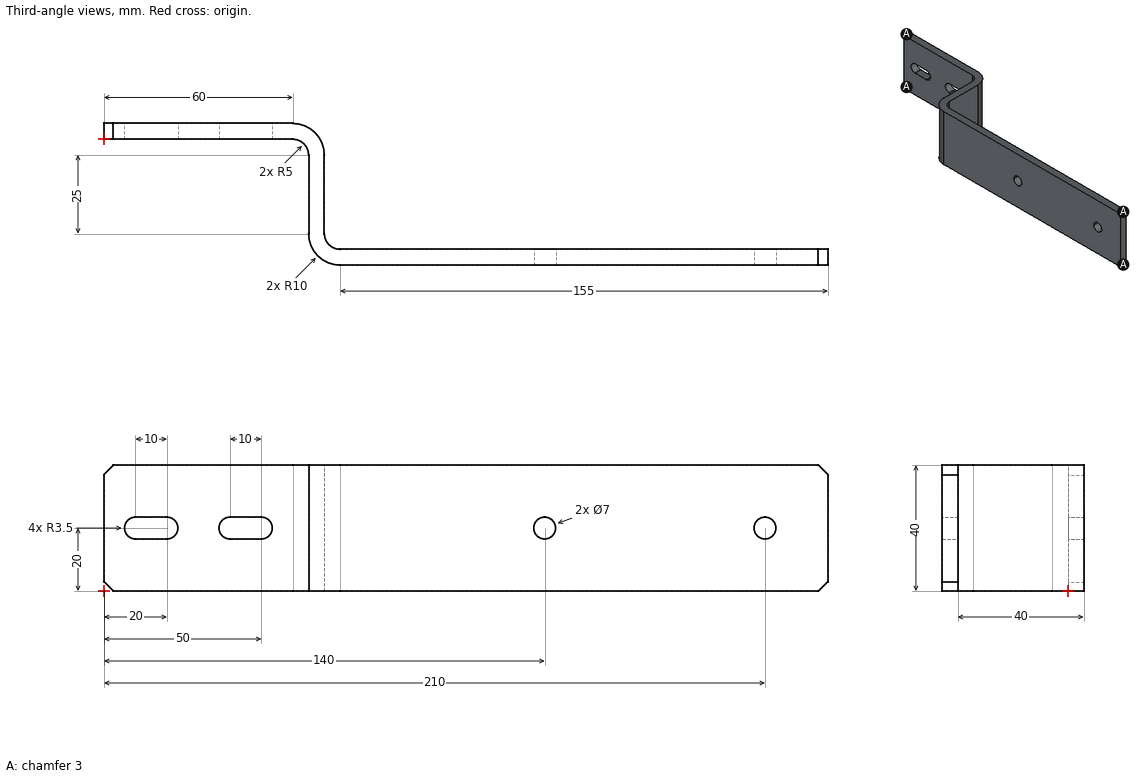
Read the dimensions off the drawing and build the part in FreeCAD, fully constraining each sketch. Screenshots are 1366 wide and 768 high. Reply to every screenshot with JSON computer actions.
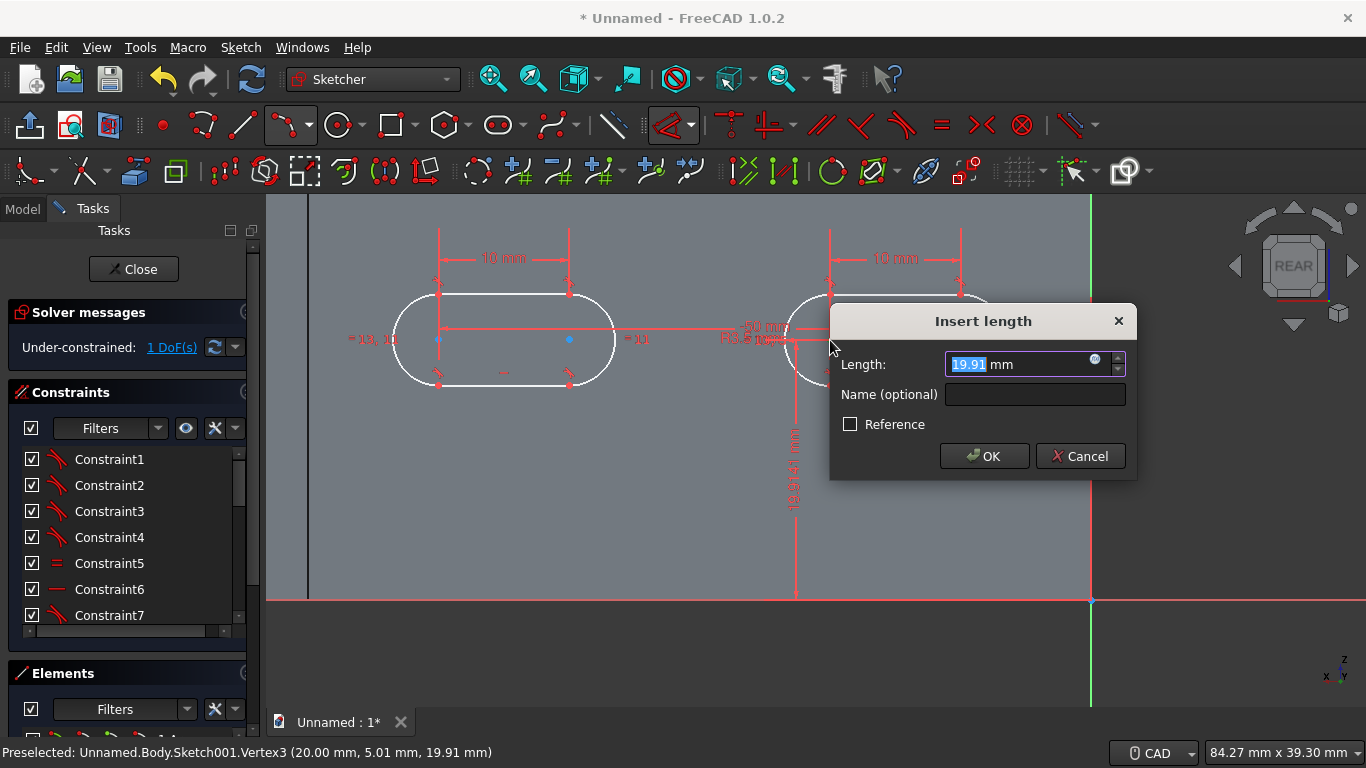
{"action": "type", "text": "20"}
{"action": "key", "text": "Return"}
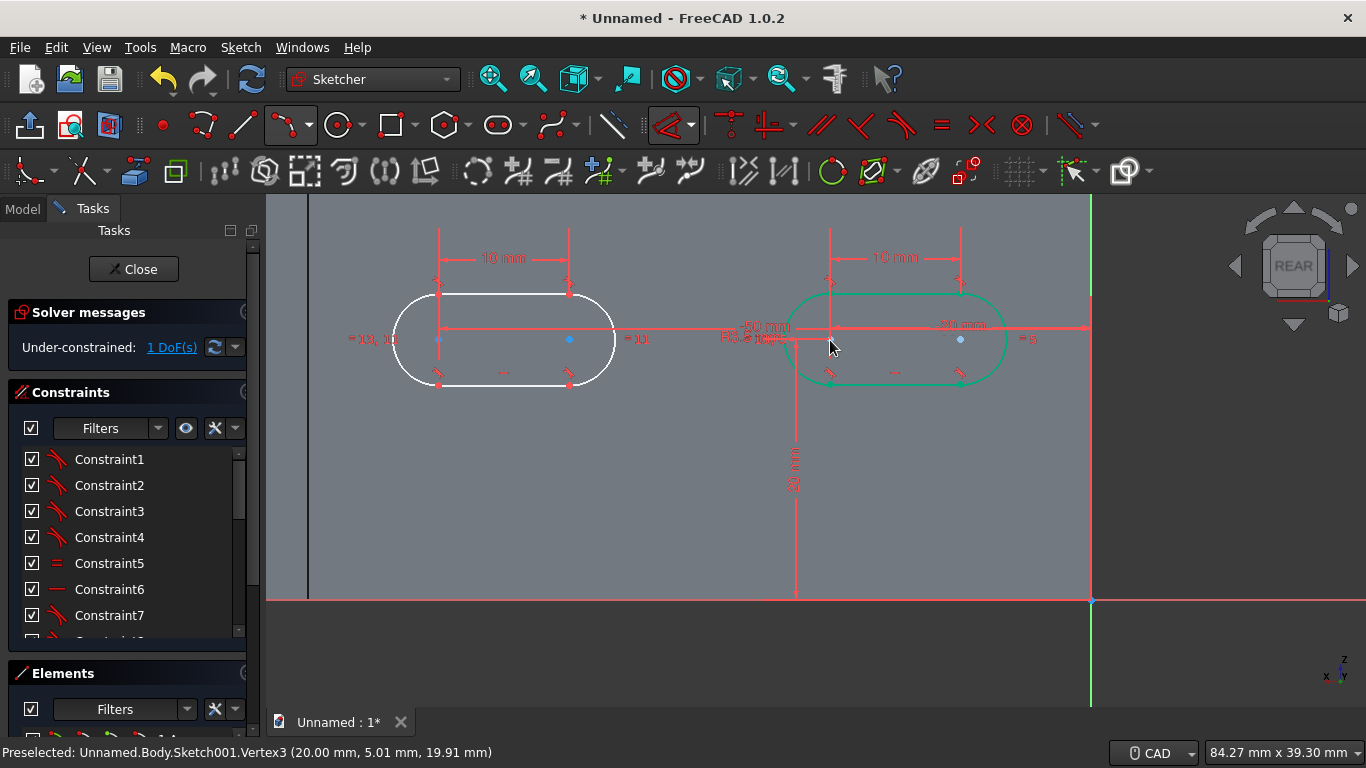
{"action": "left_click", "coordinate": [439, 340]}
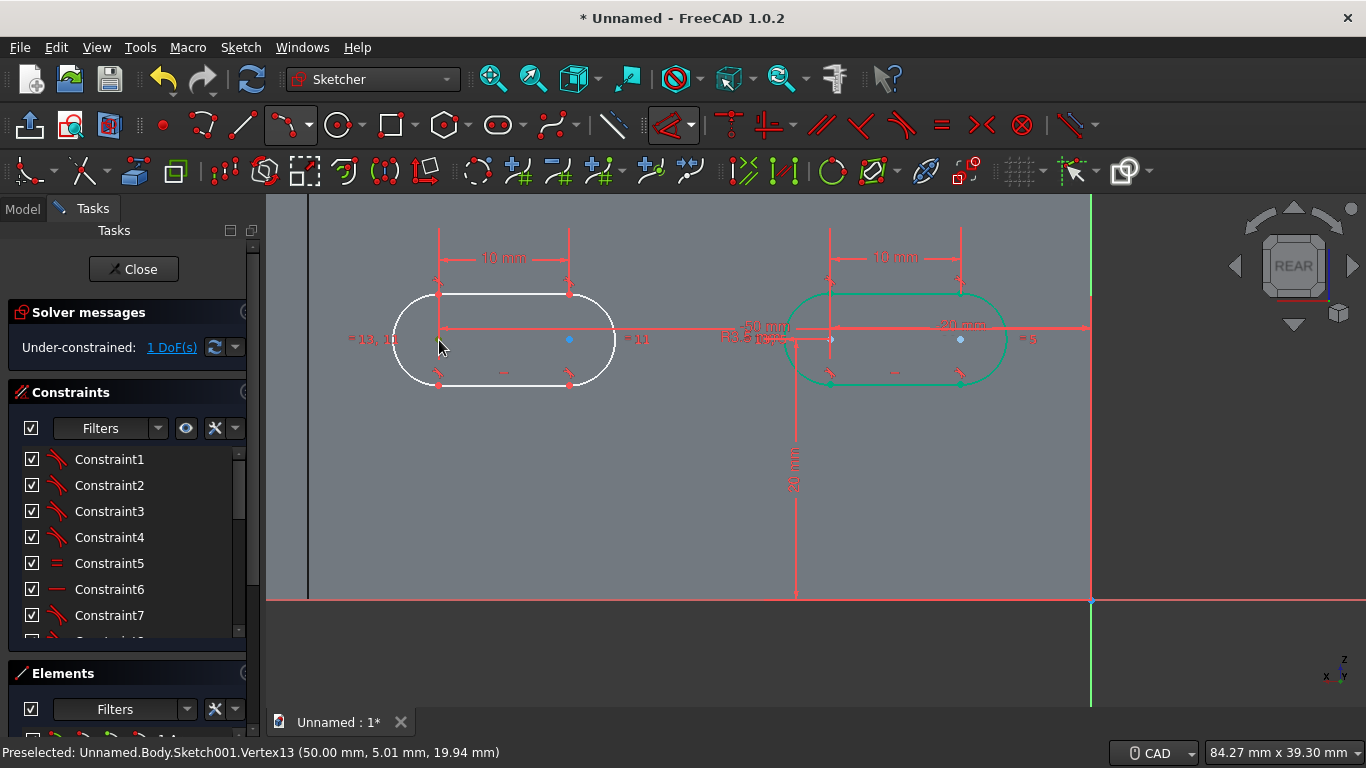
{"action": "key", "text": "i"}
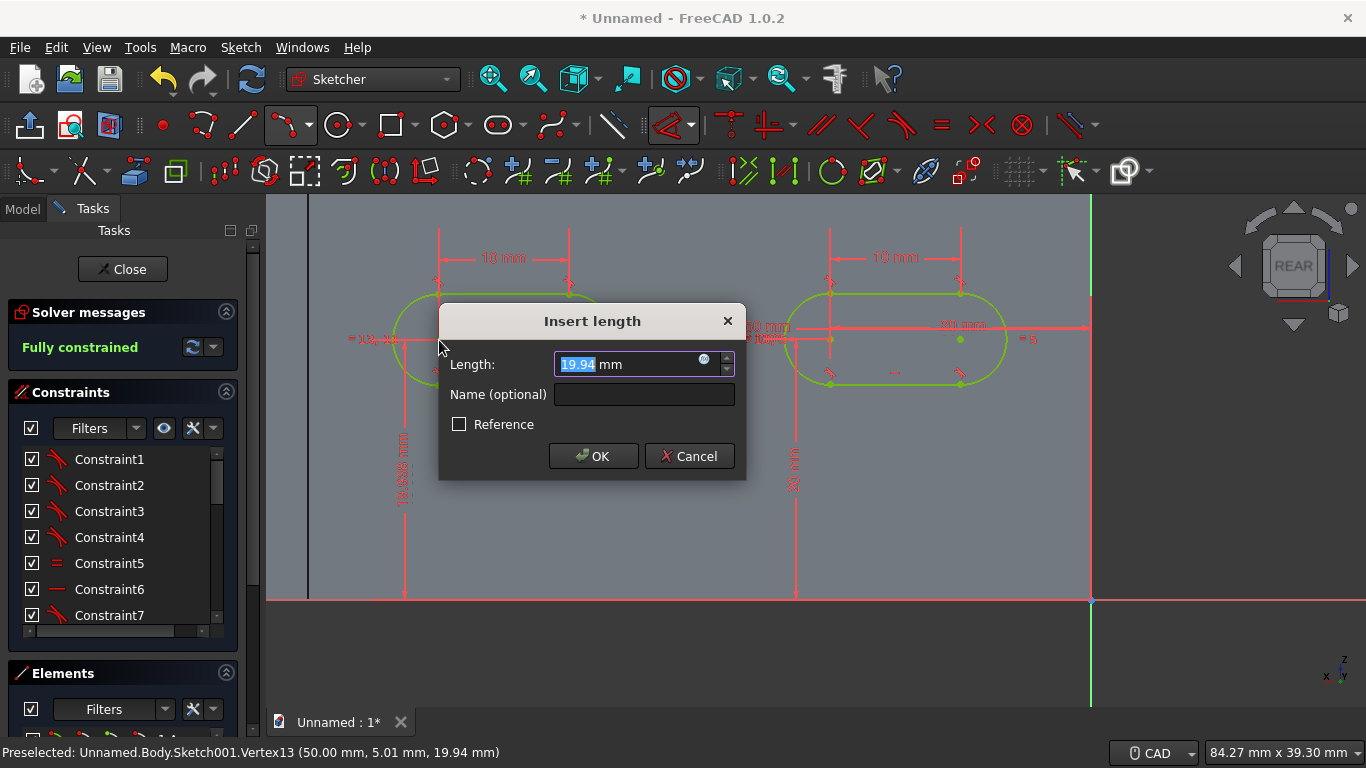
{"action": "type", "text": "20"}
{"action": "key", "text": "Return"}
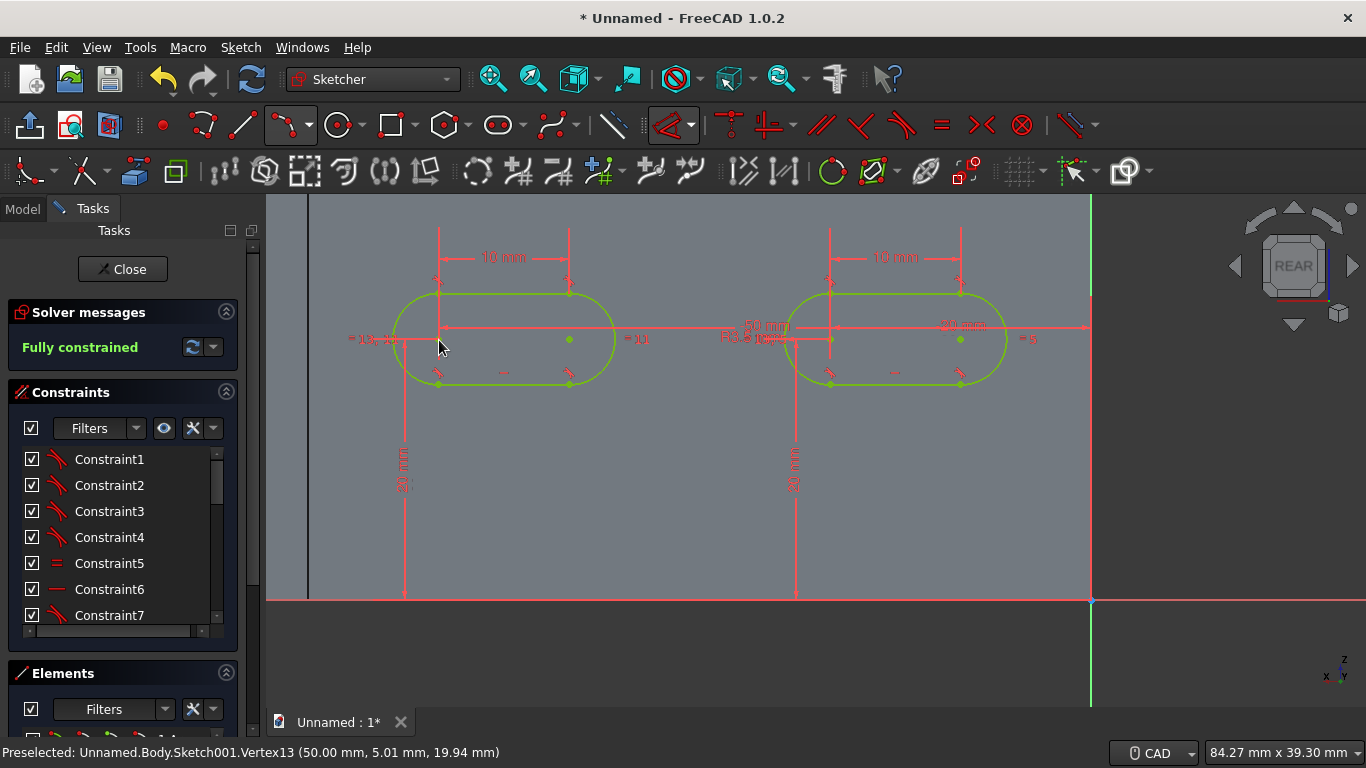
{"action": "left_click", "coordinate": [123, 269]}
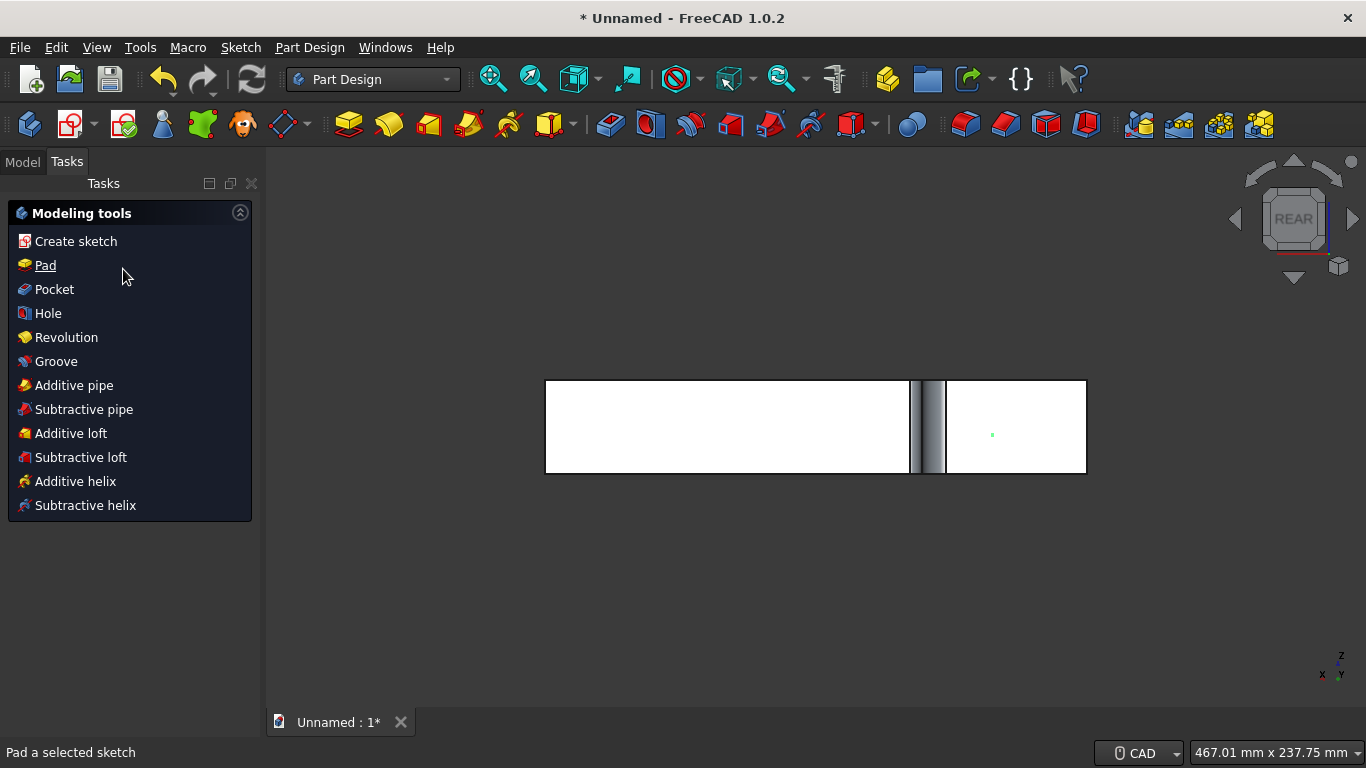
{"action": "left_click", "coordinate": [612, 124]}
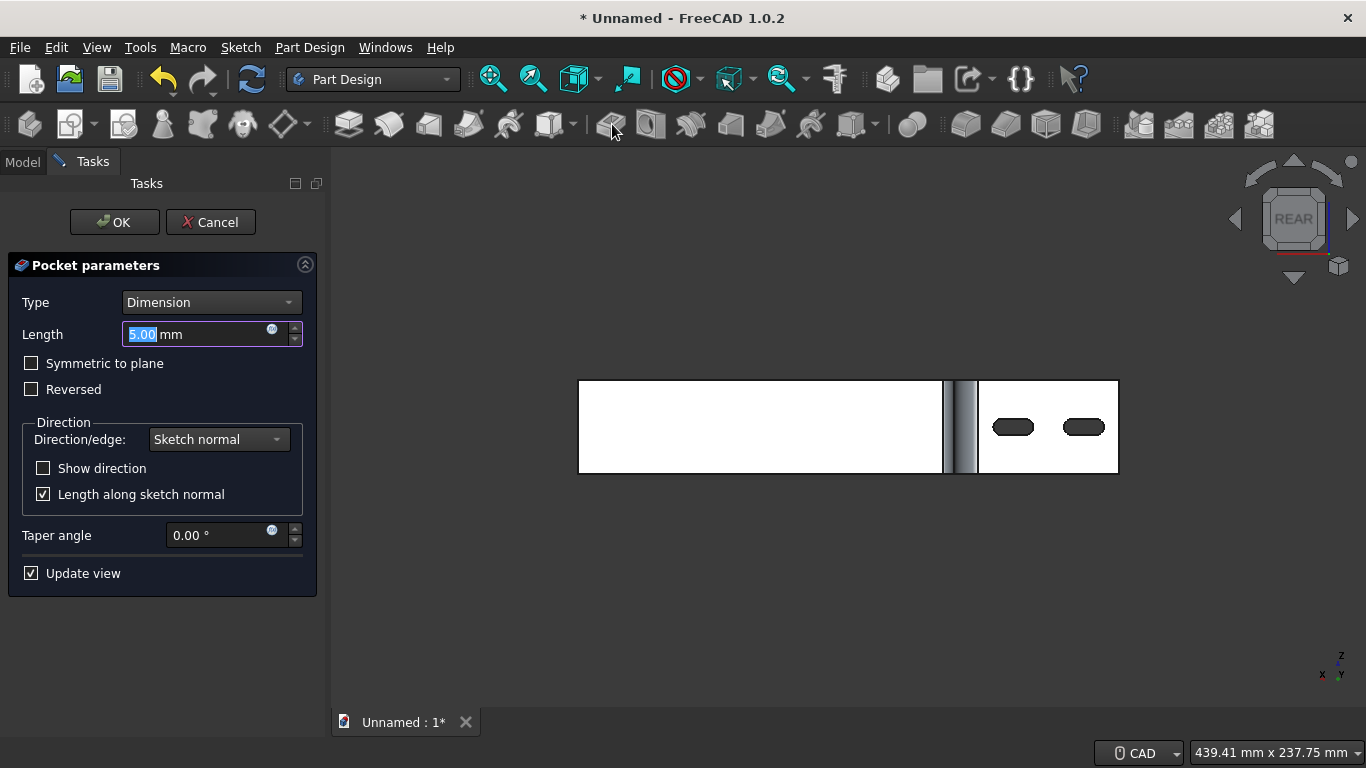
{"action": "type", "text": "40"}
{"action": "key", "text": "Tab"}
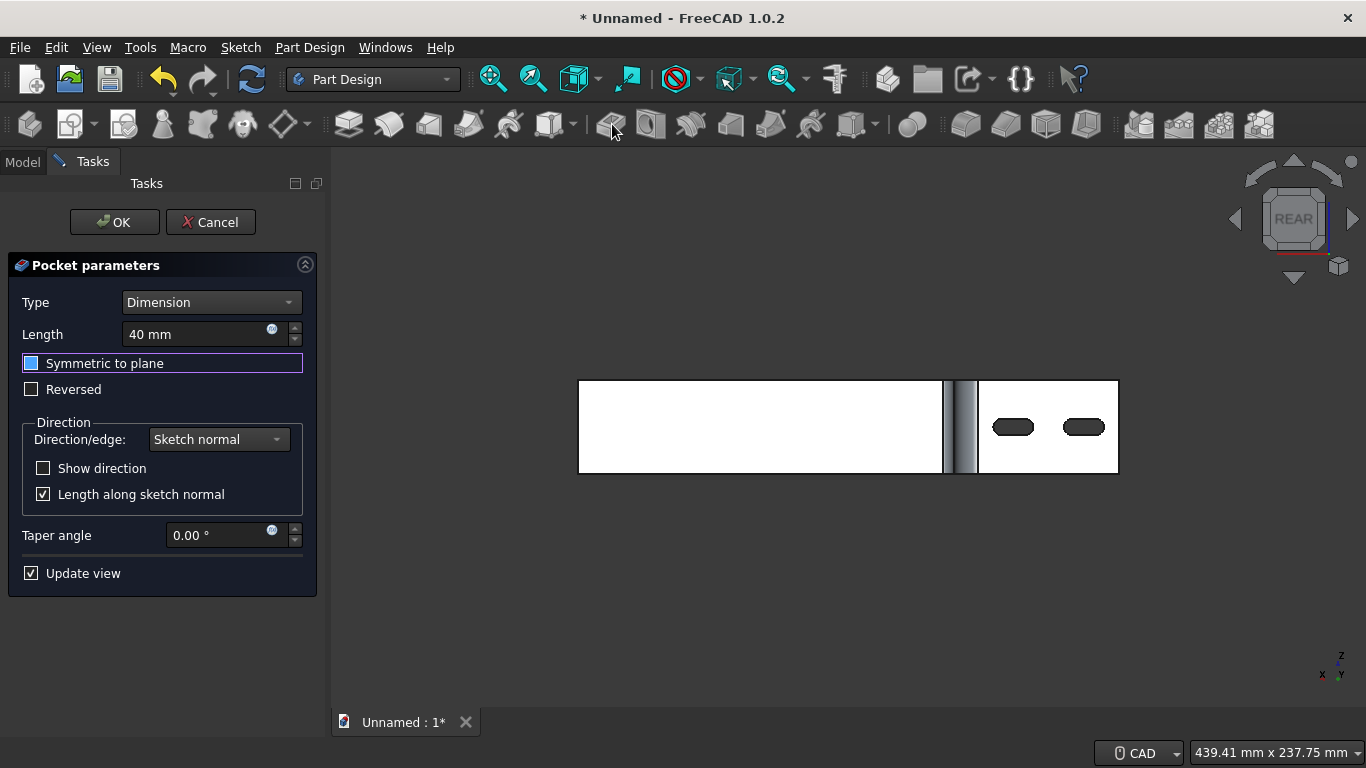
{"action": "left_click", "coordinate": [115, 222]}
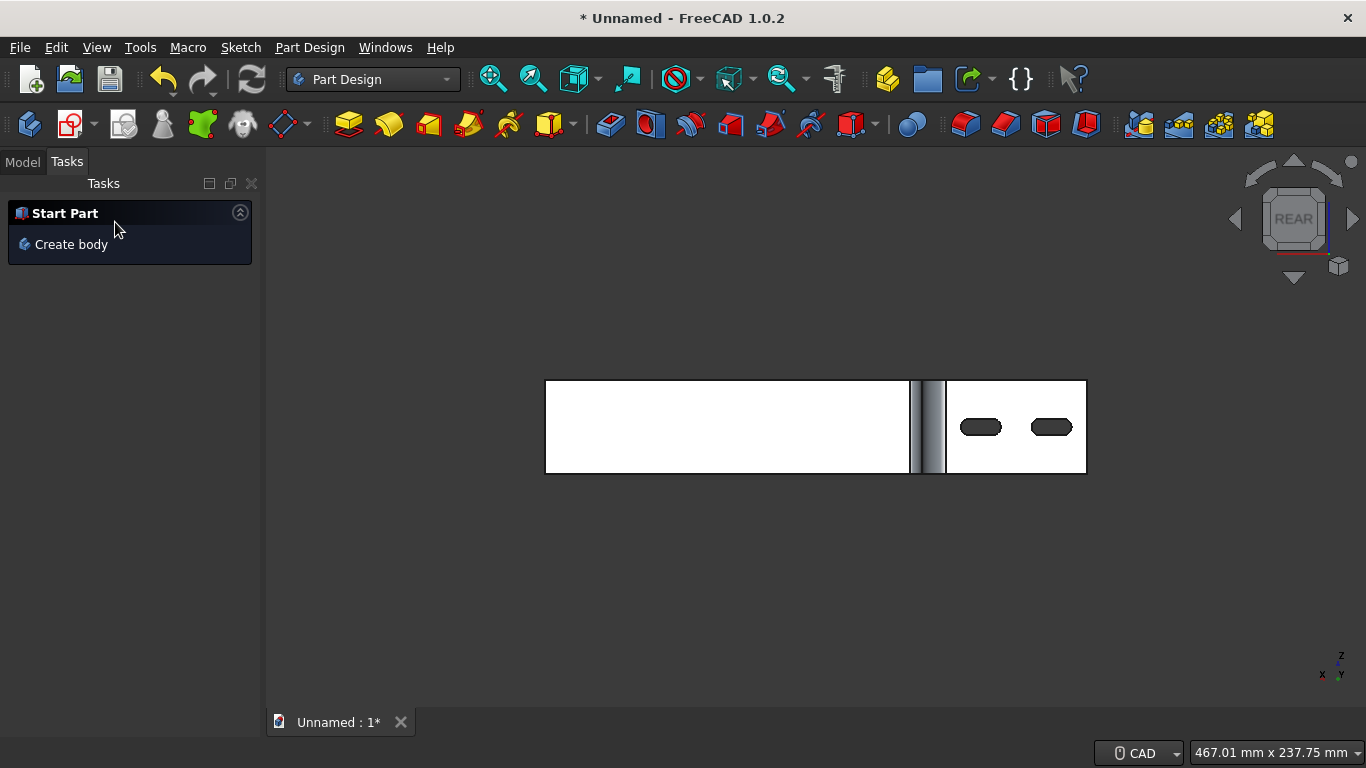
{"action": "left_click", "coordinate": [623, 426]}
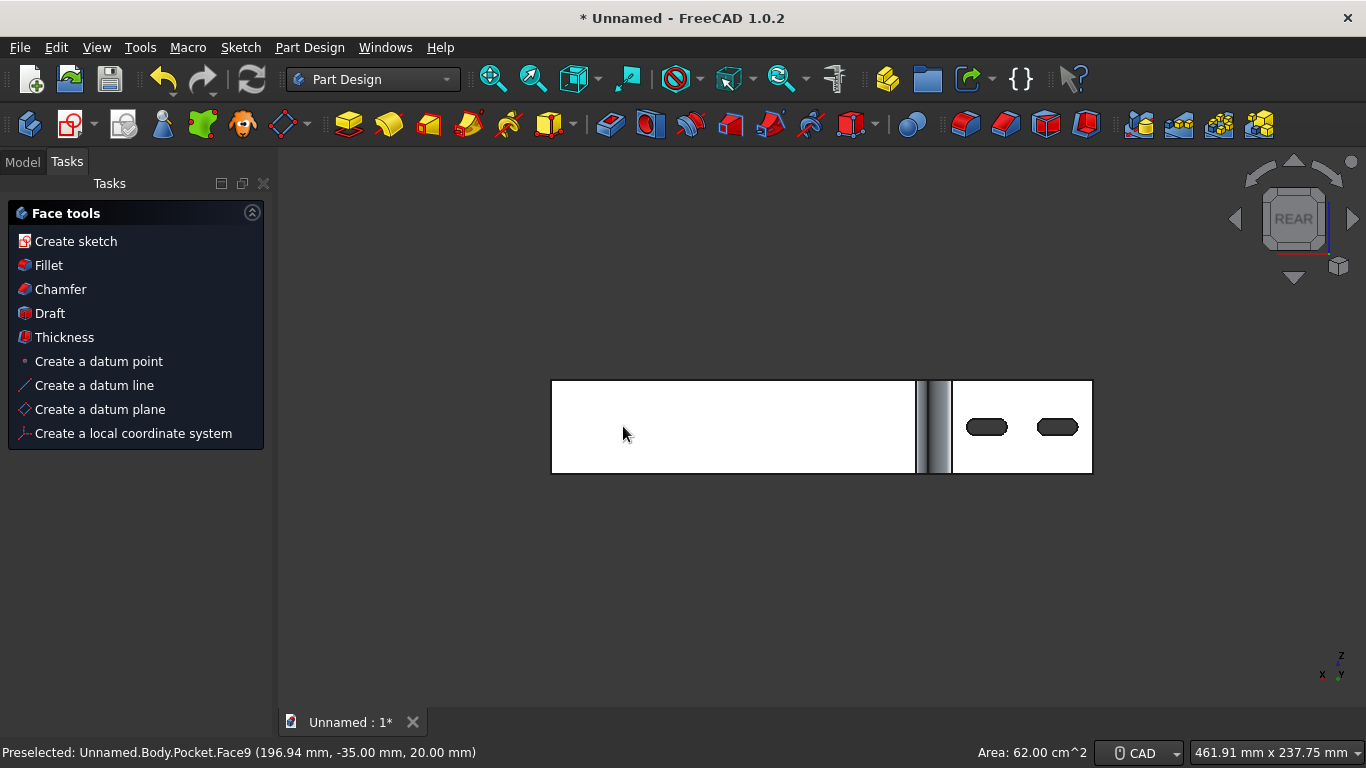
{"action": "left_click", "coordinate": [70, 124]}